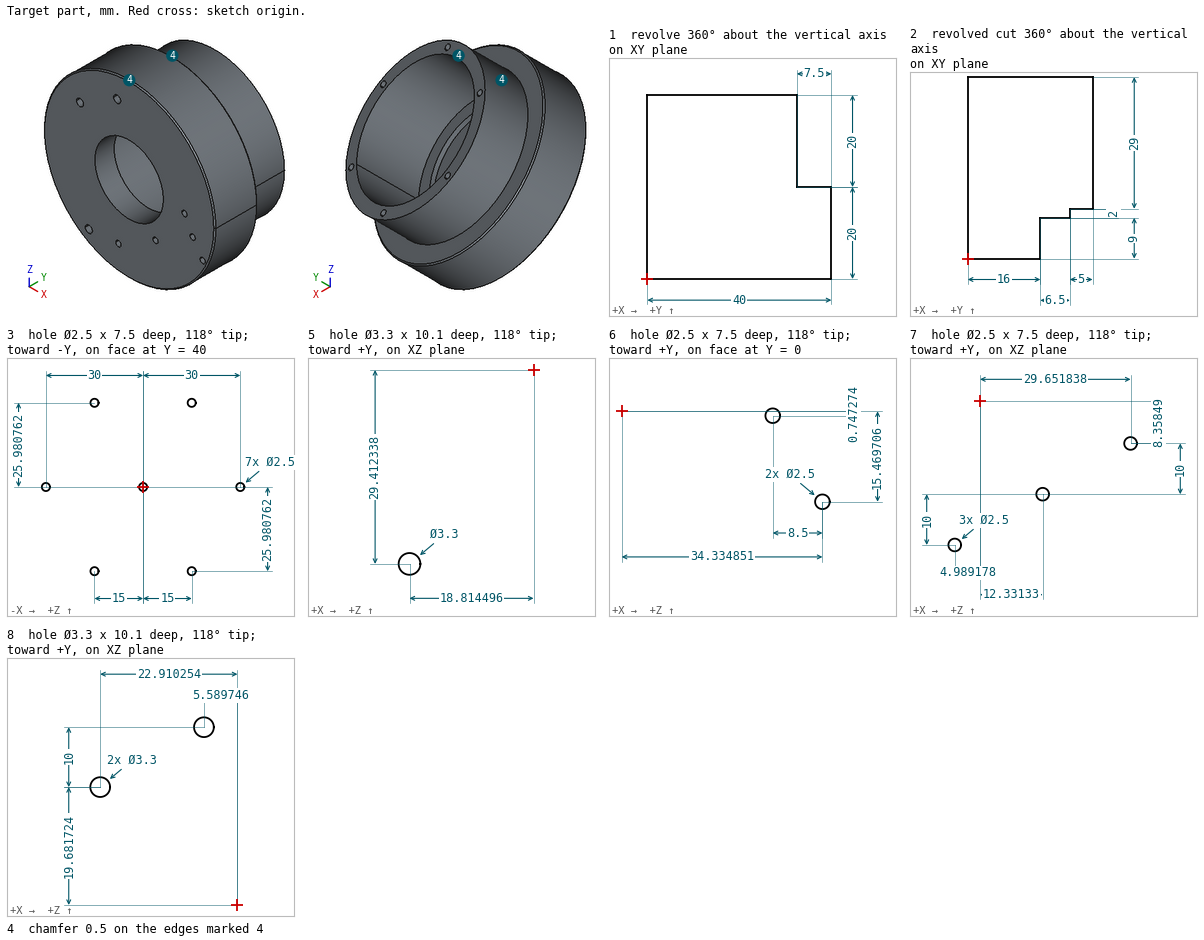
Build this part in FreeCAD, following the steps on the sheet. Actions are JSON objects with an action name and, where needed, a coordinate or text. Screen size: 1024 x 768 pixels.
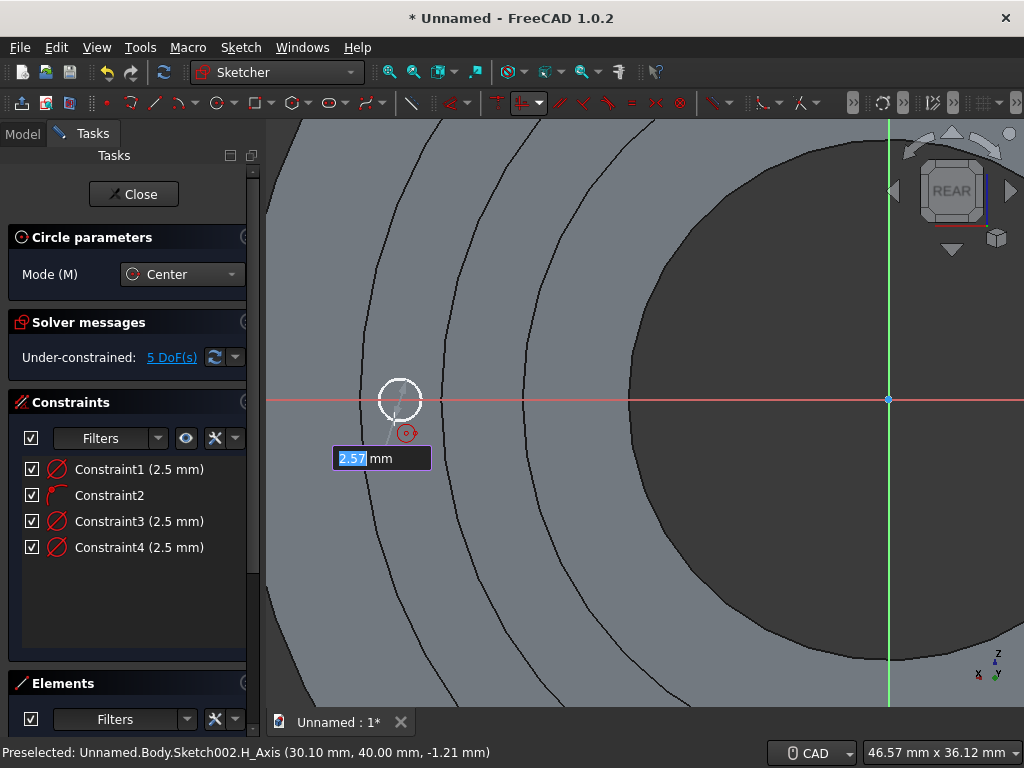
{"action": "type", "text": "2.5"}
{"action": "key", "text": "Return"}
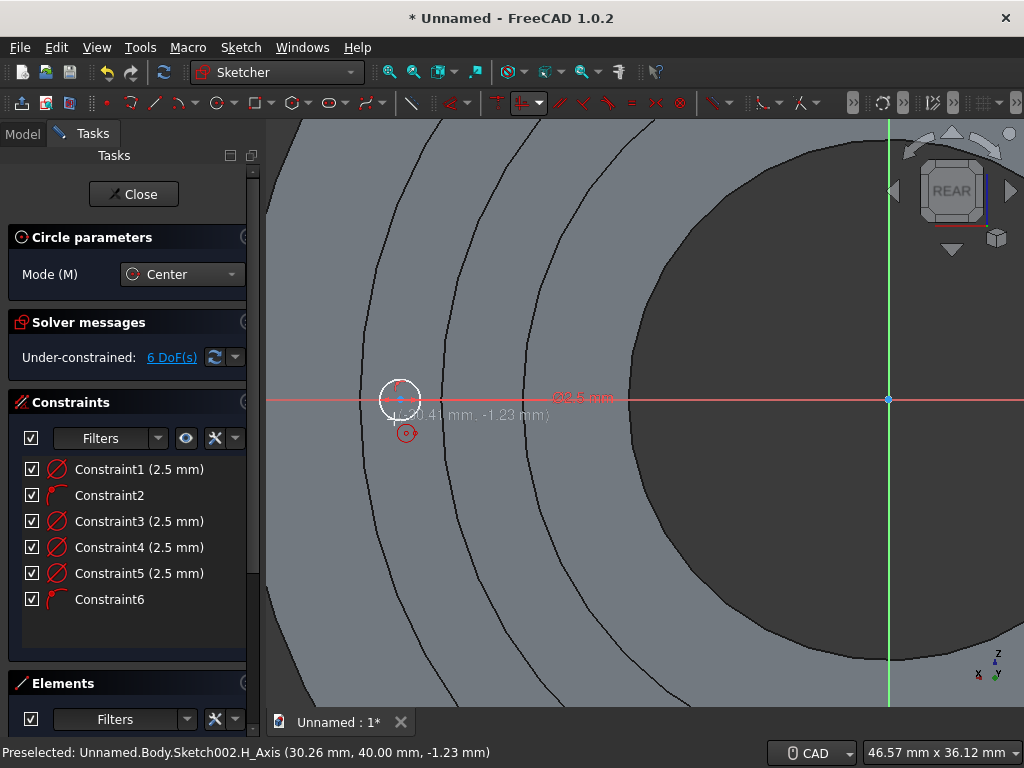
{"action": "scroll", "coordinate": [395, 421], "scroll_direction": "down", "scroll_amount": 5}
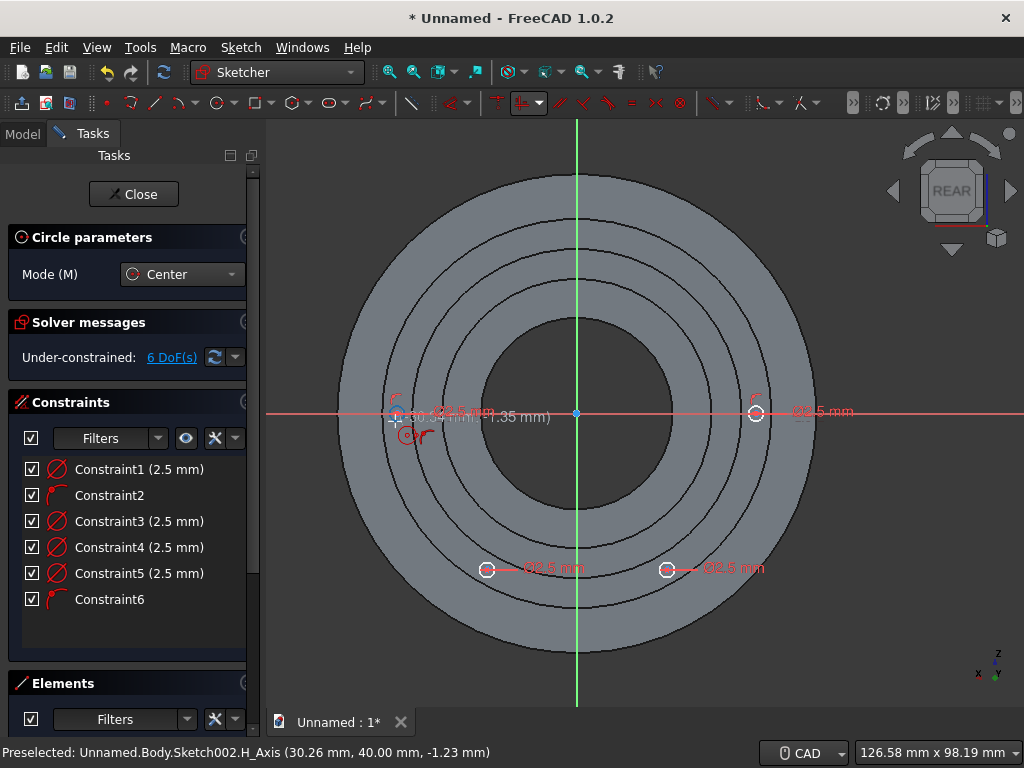
{"action": "scroll", "coordinate": [487, 258], "scroll_direction": "up", "scroll_amount": 6}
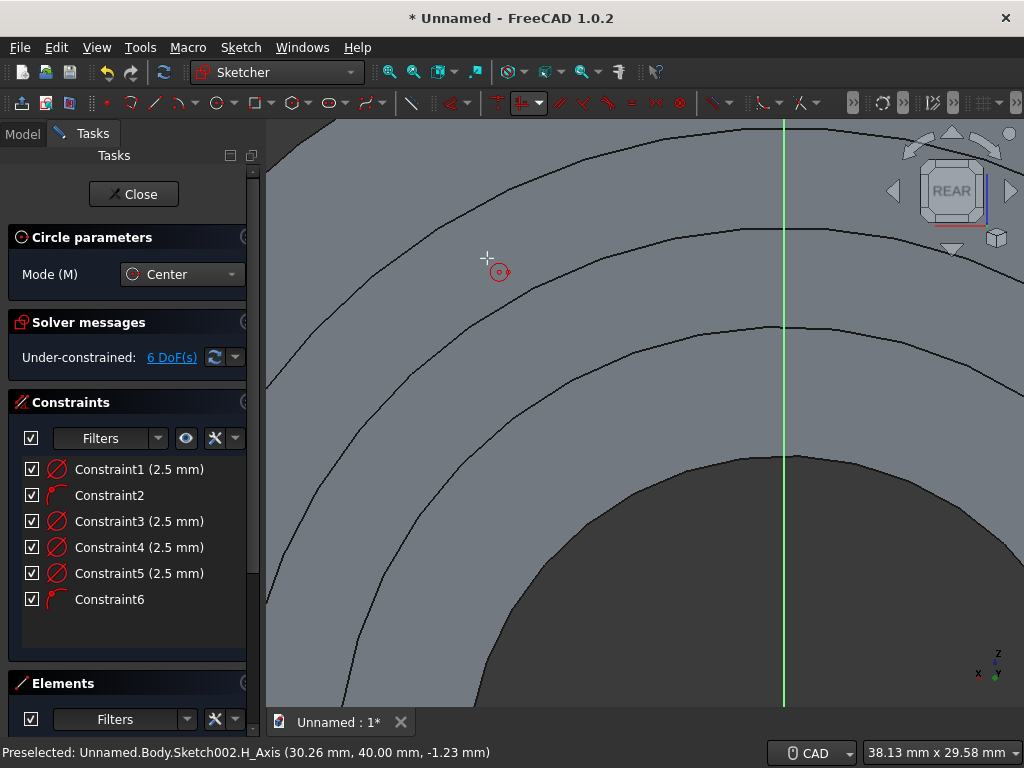
{"action": "scroll", "coordinate": [487, 257], "scroll_direction": "down", "scroll_amount": 6}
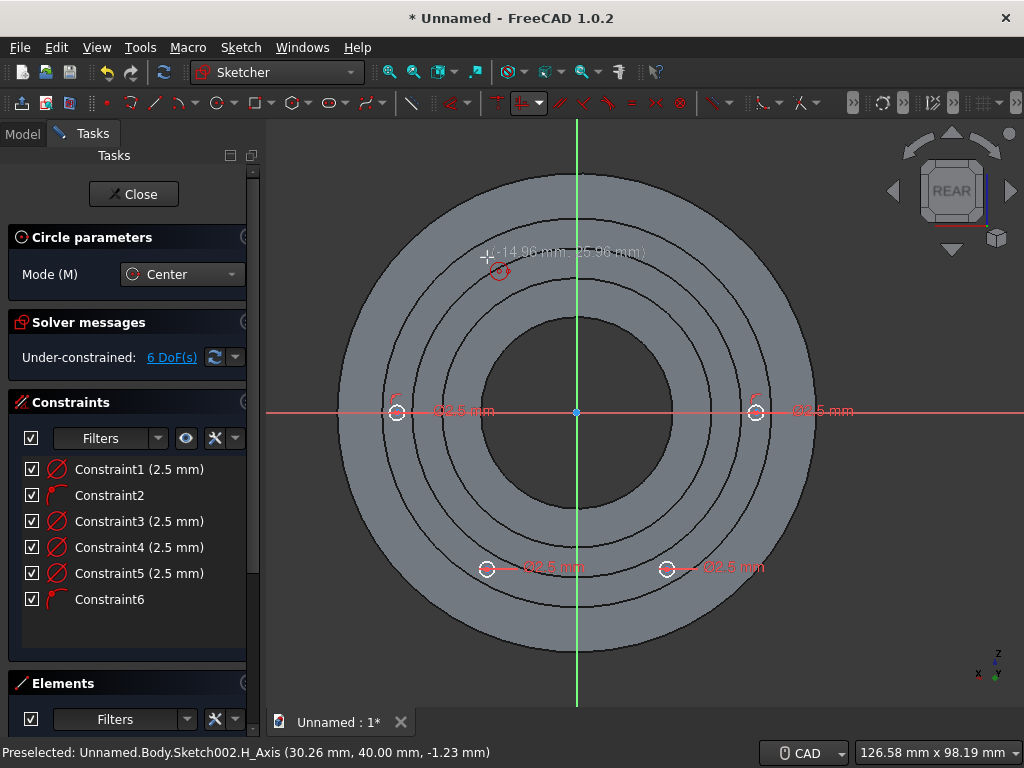
{"action": "left_click", "coordinate": [487, 257]}
{"action": "mouse_move", "coordinate": [492, 252]}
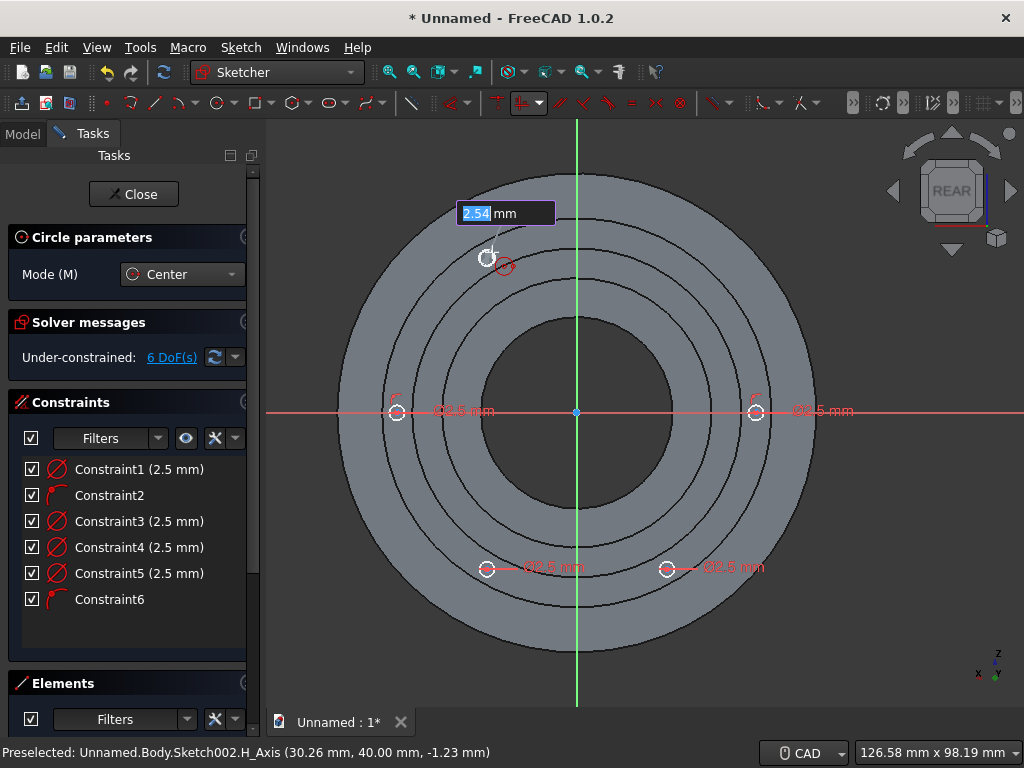
{"action": "type", "text": "2.5"}
{"action": "key", "text": "Return"}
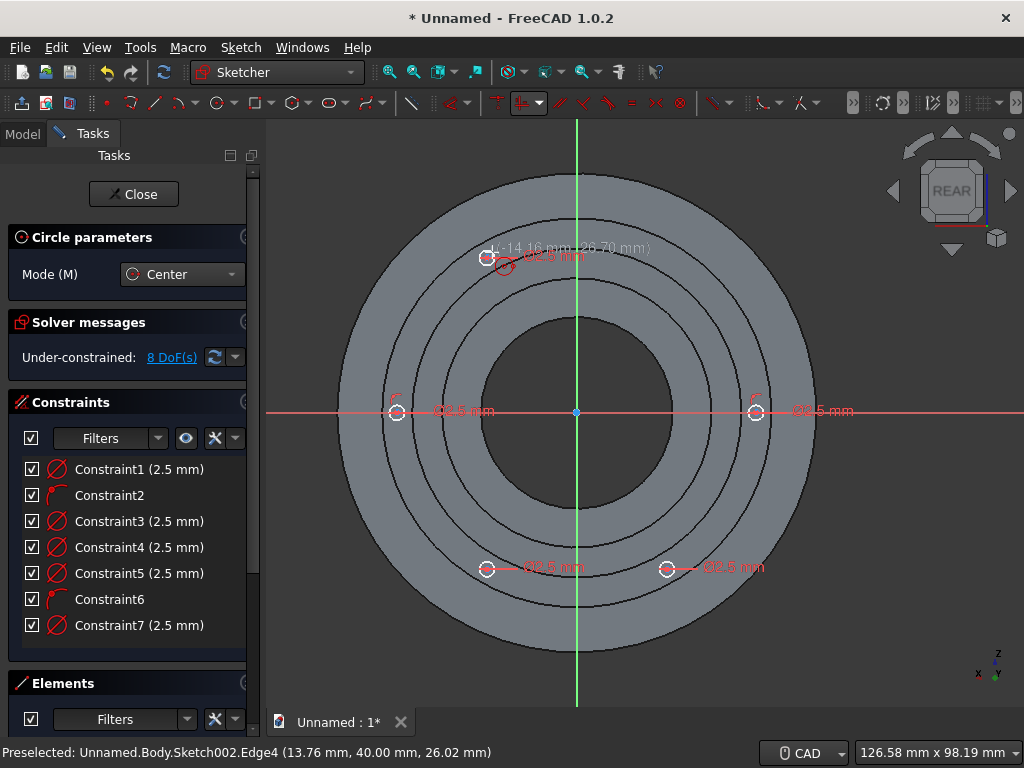
{"action": "scroll", "coordinate": [667, 257], "scroll_direction": "up", "scroll_amount": 6}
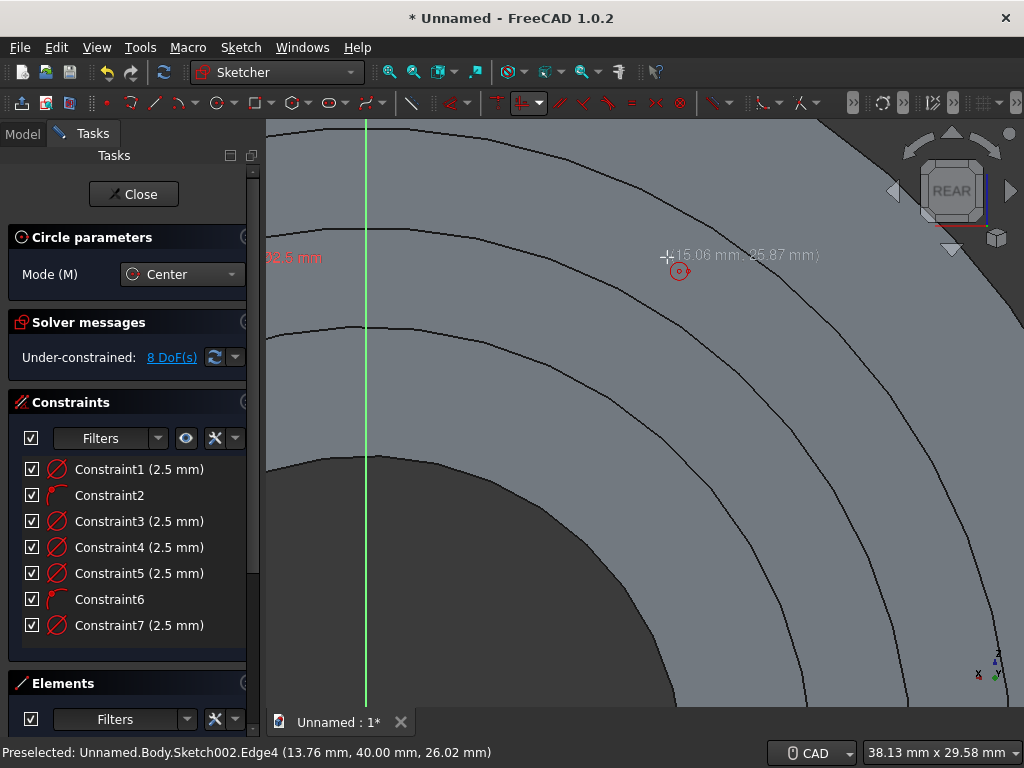
{"action": "scroll", "coordinate": [667, 257], "scroll_direction": "down", "scroll_amount": 6}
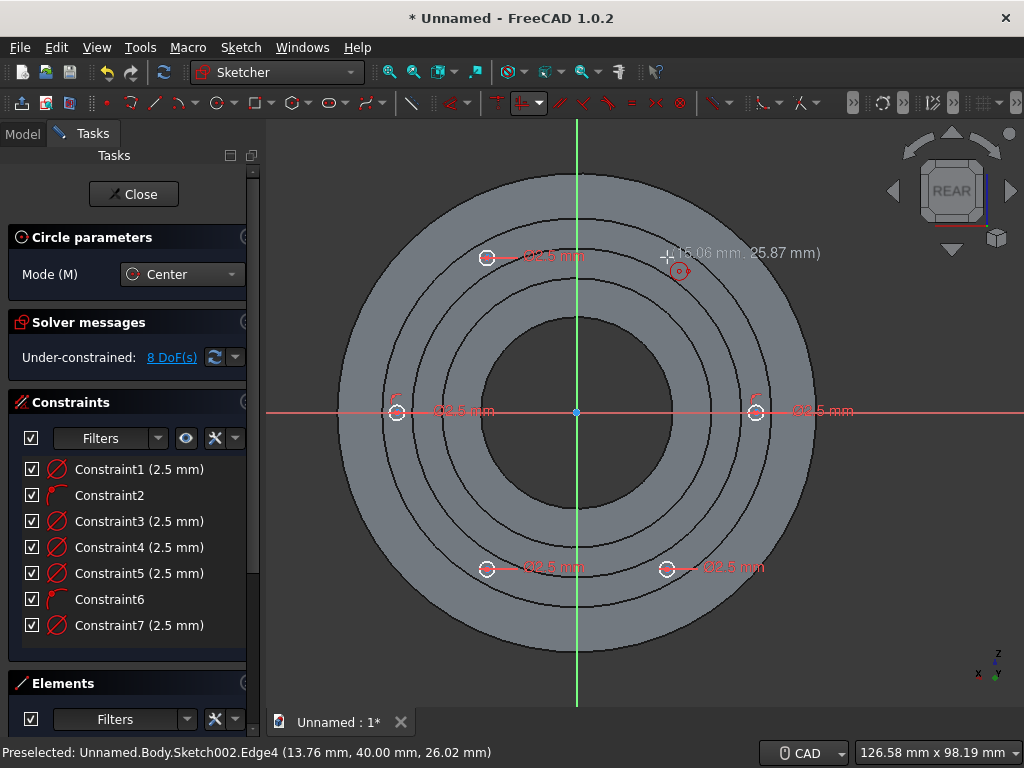
{"action": "left_click", "coordinate": [667, 257]}
{"action": "mouse_move", "coordinate": [672, 252]}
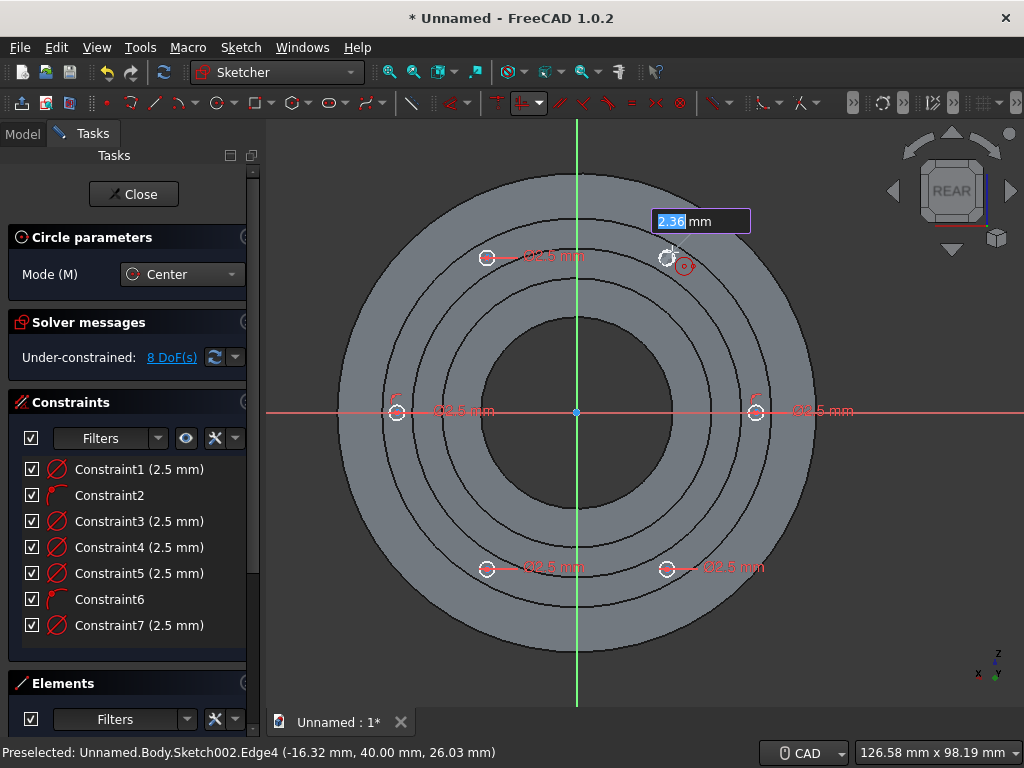
{"action": "type", "text": "2.5"}
{"action": "key", "text": "Return"}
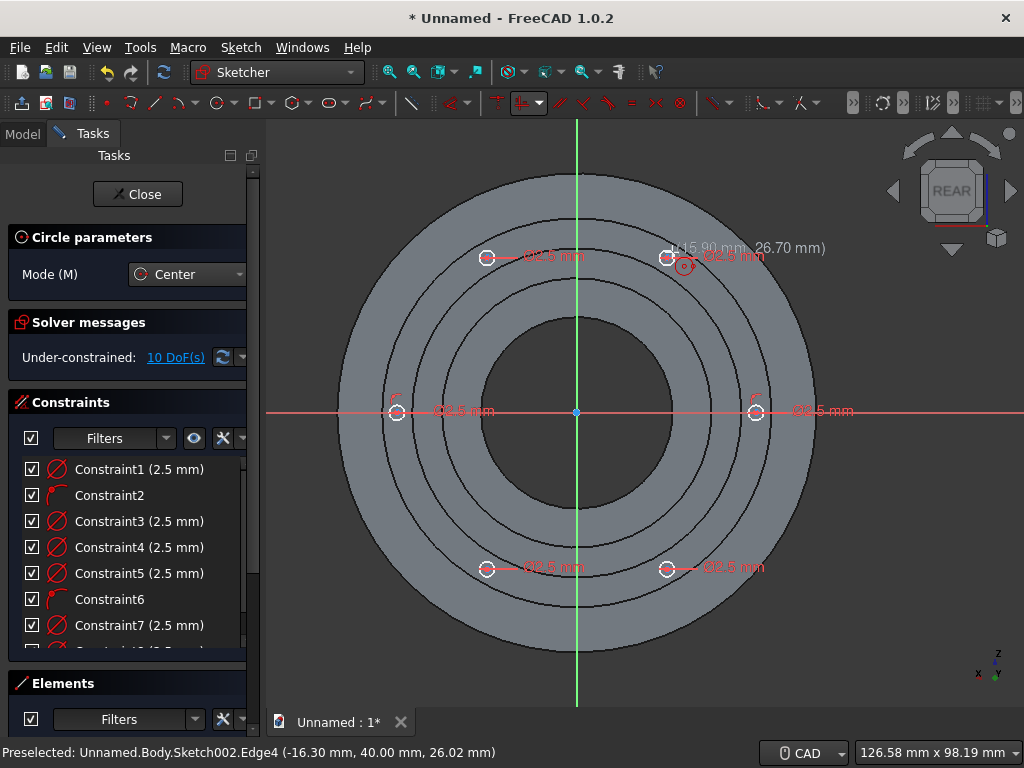
{"action": "scroll", "coordinate": [577, 413], "scroll_direction": "up", "scroll_amount": 6}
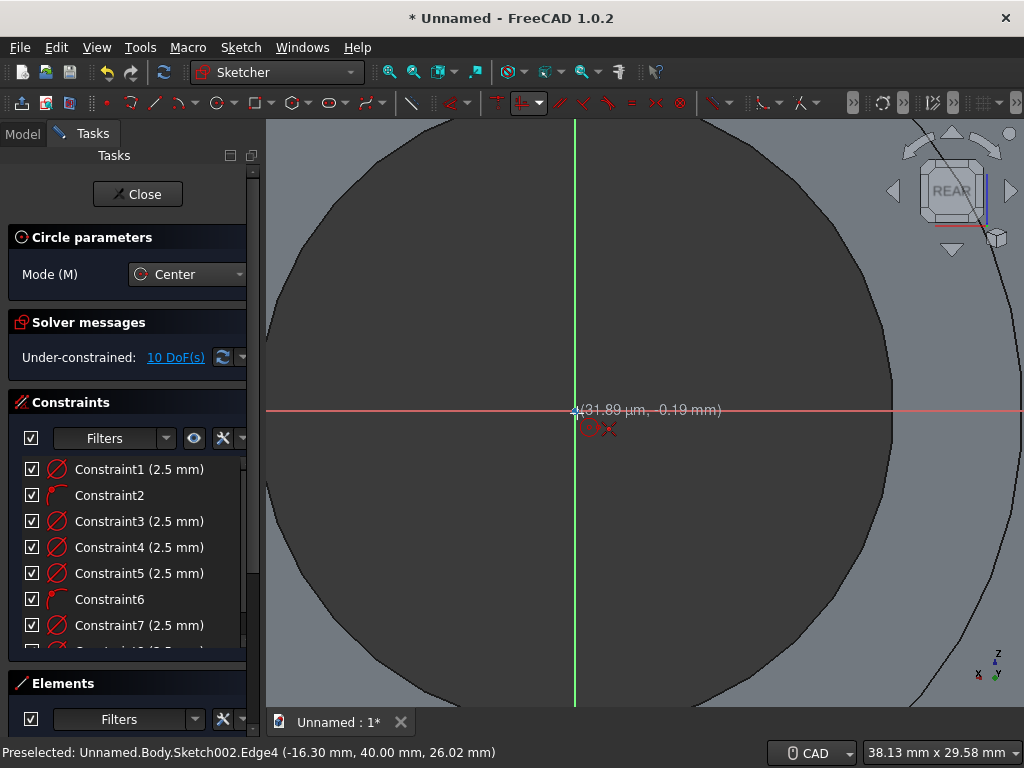
{"action": "scroll", "coordinate": [577, 414], "scroll_direction": "down", "scroll_amount": 6}